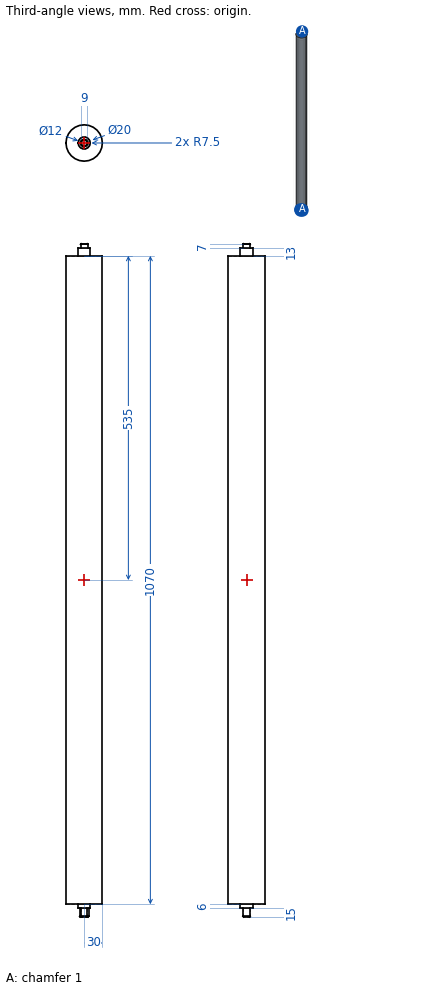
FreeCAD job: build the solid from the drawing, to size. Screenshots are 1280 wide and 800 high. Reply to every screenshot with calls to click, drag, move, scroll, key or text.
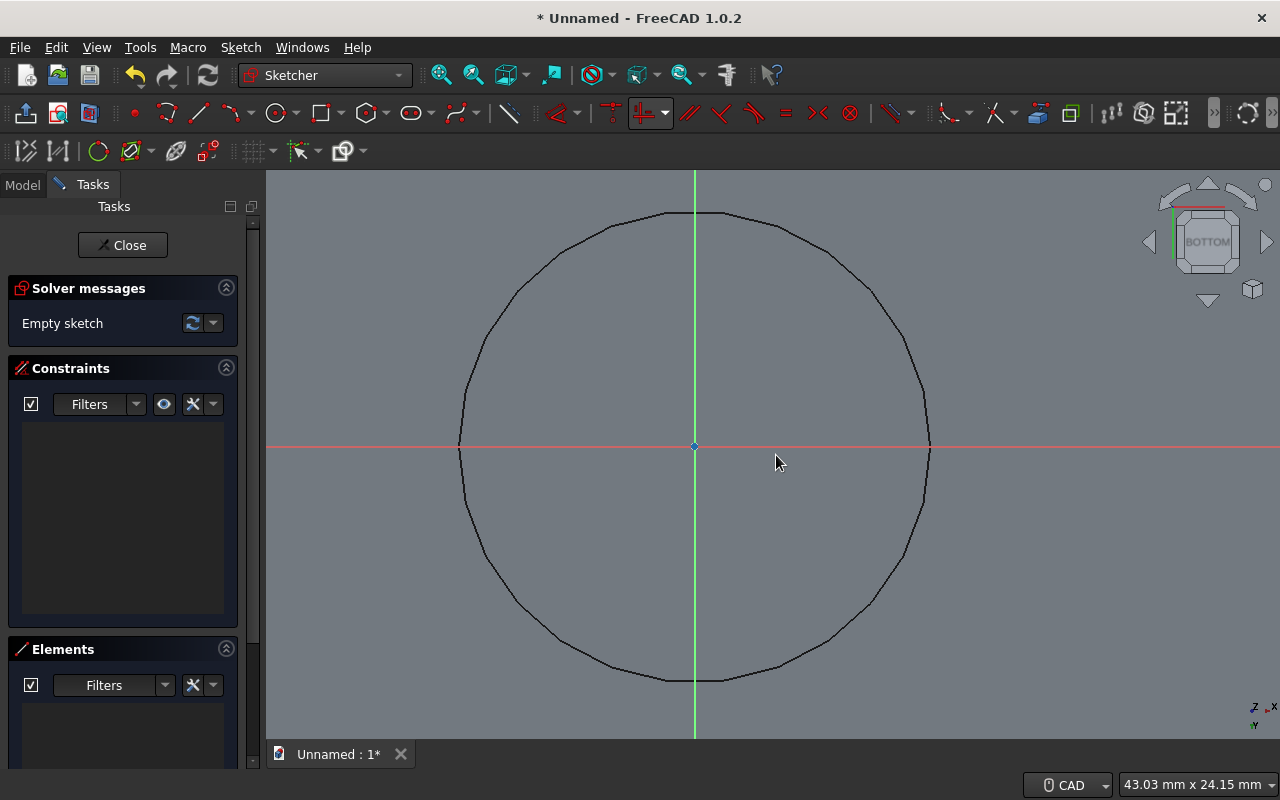
key(g)
key(l)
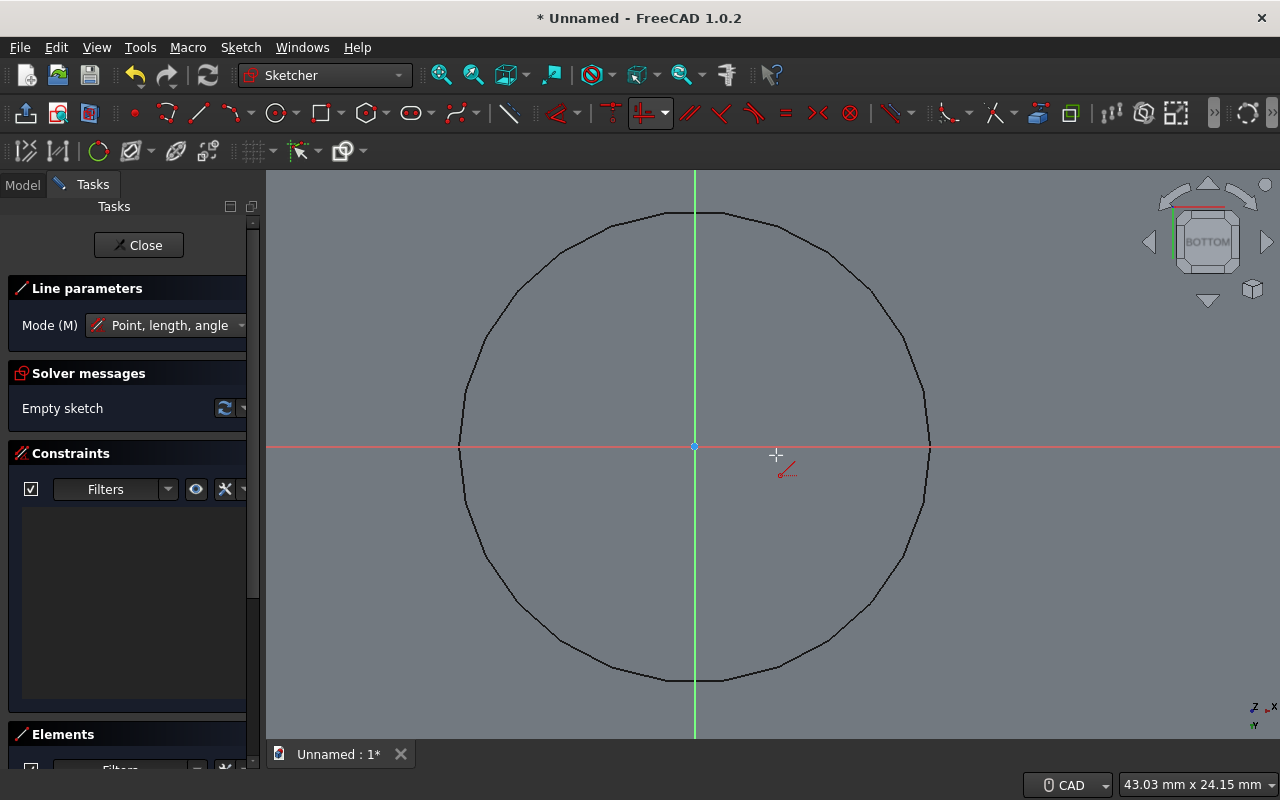
click(589, 588)
click(801, 588)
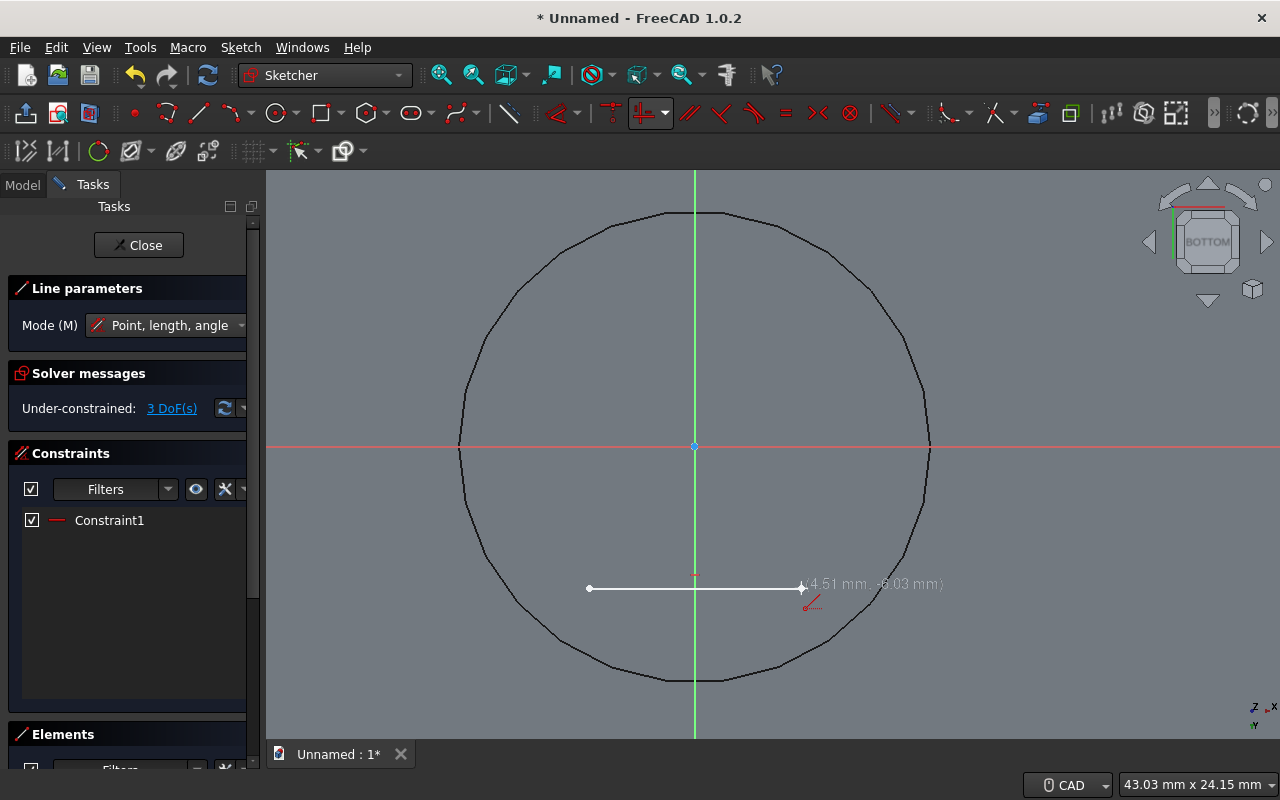
click(801, 306)
click(589, 306)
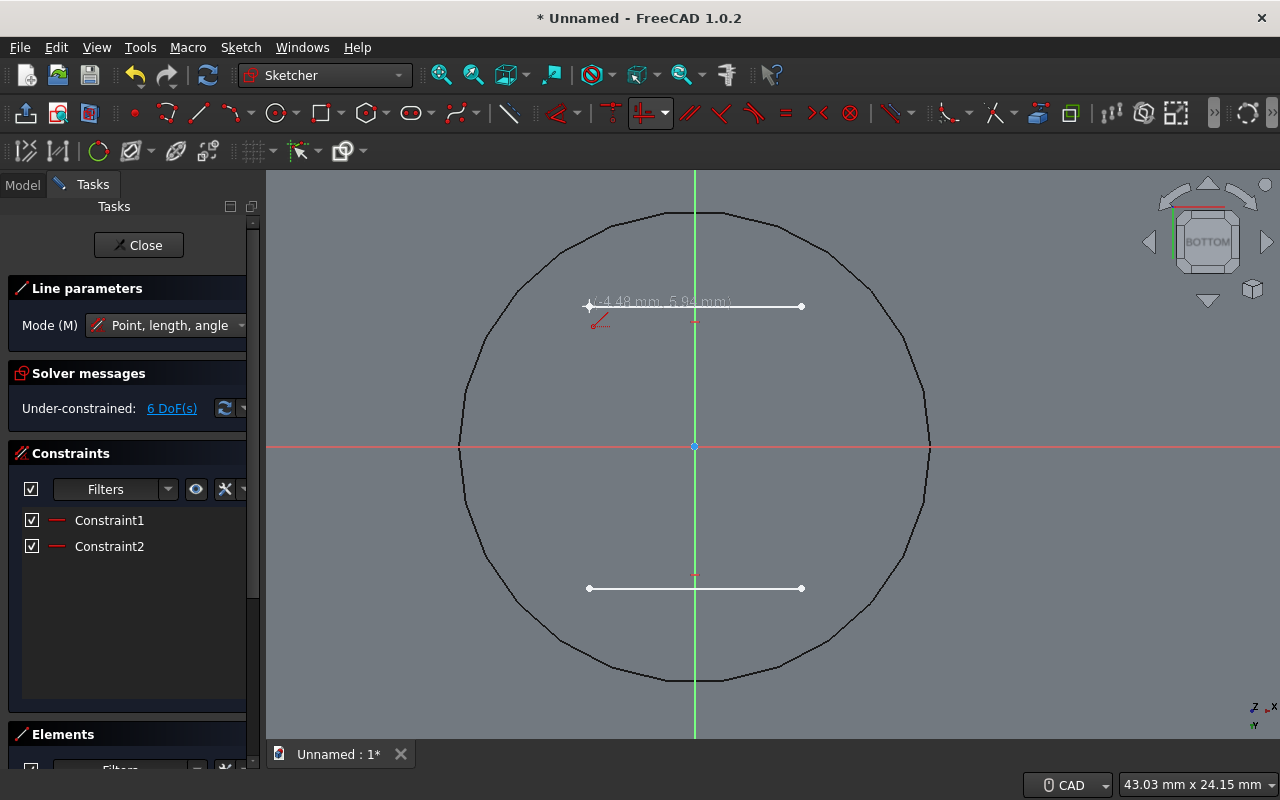
key(g)
key(3)
key(a)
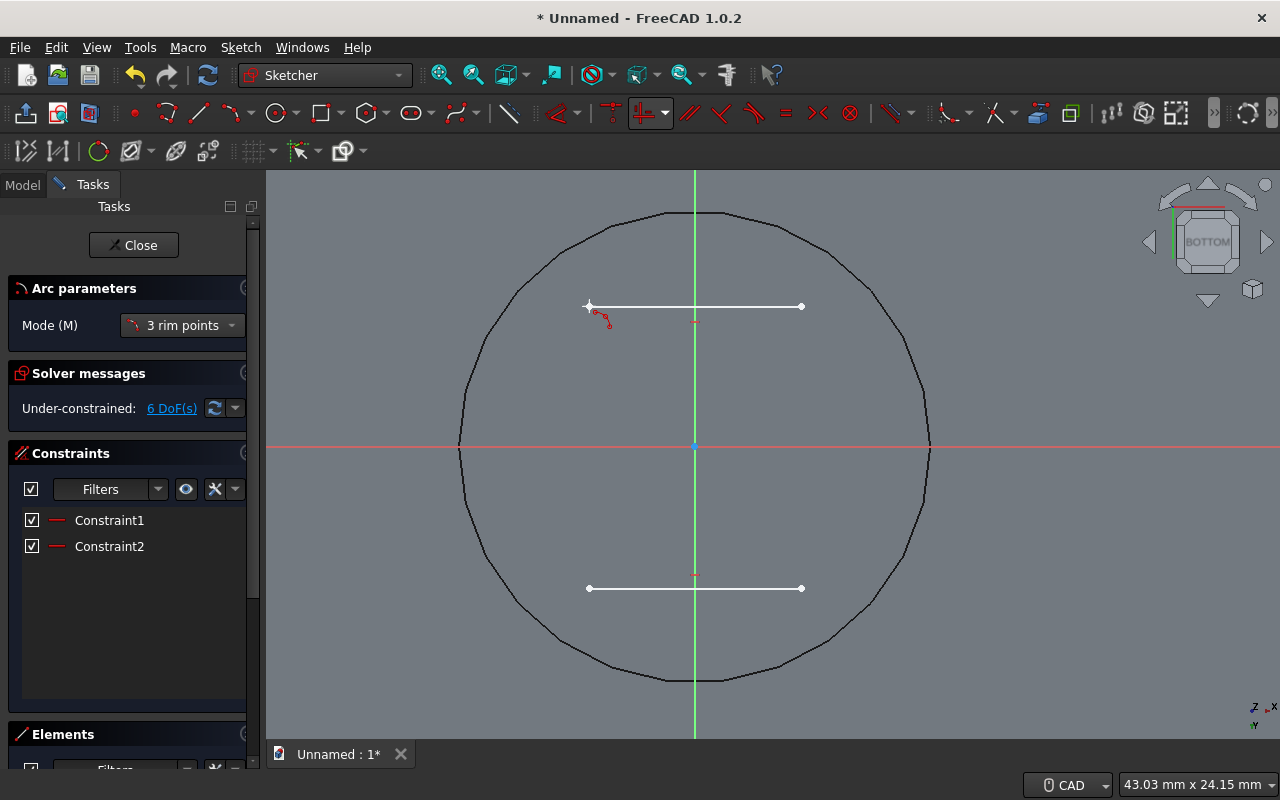
click(801, 589)
click(801, 307)
click(868, 480)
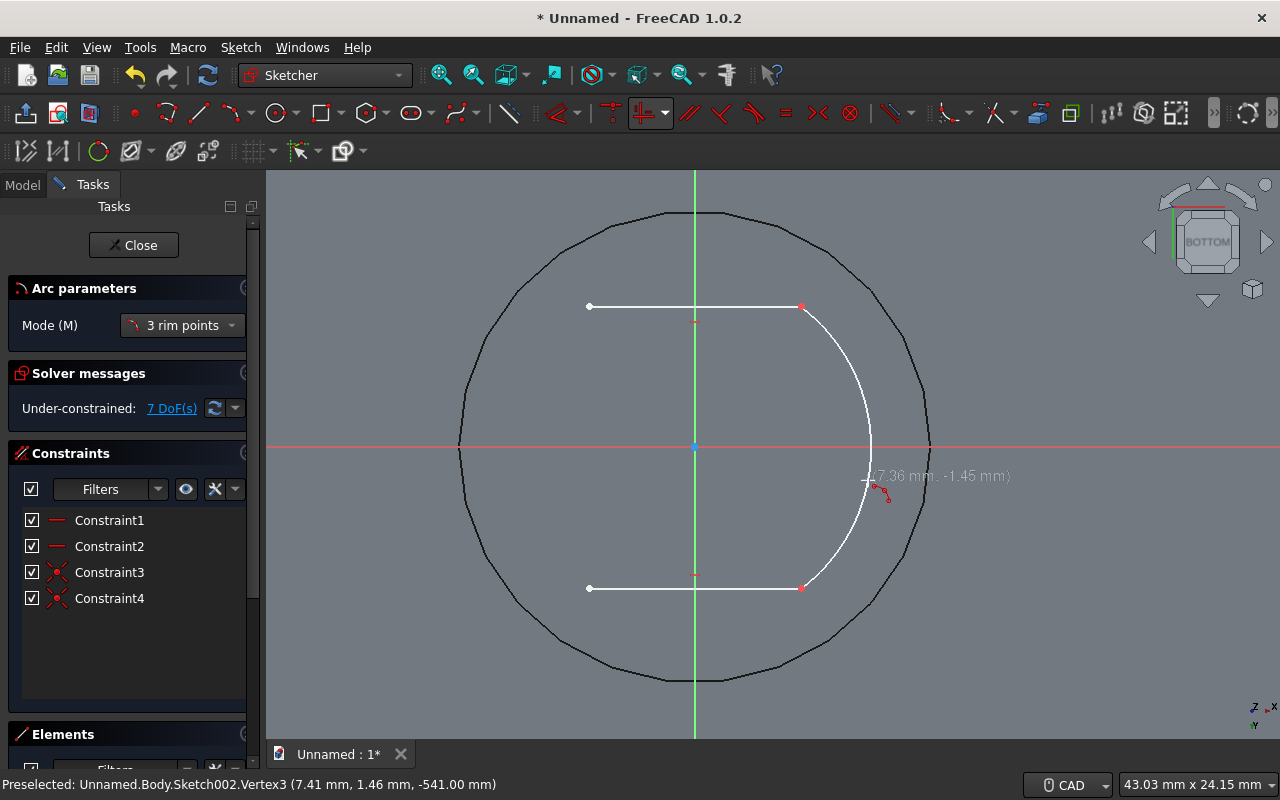
click(589, 307)
click(589, 589)
click(521, 414)
key(Escape)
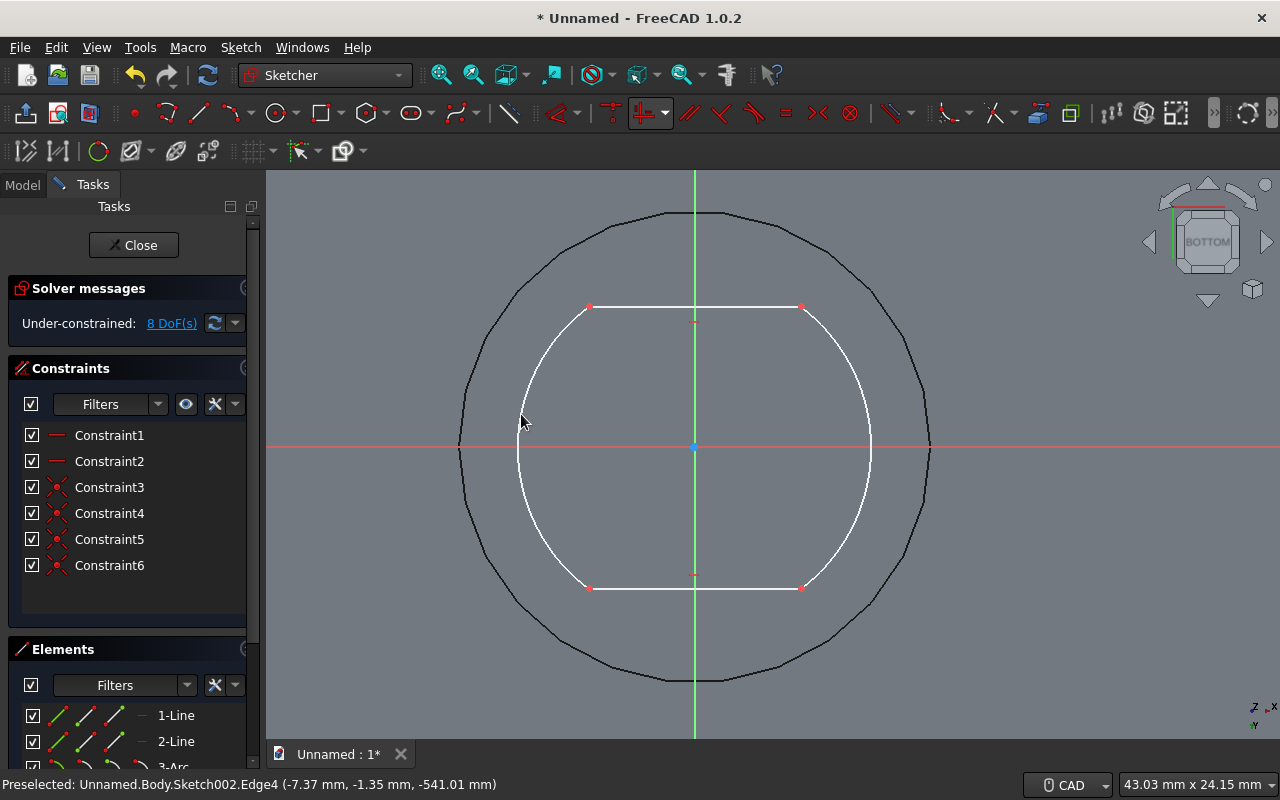
click(859, 512)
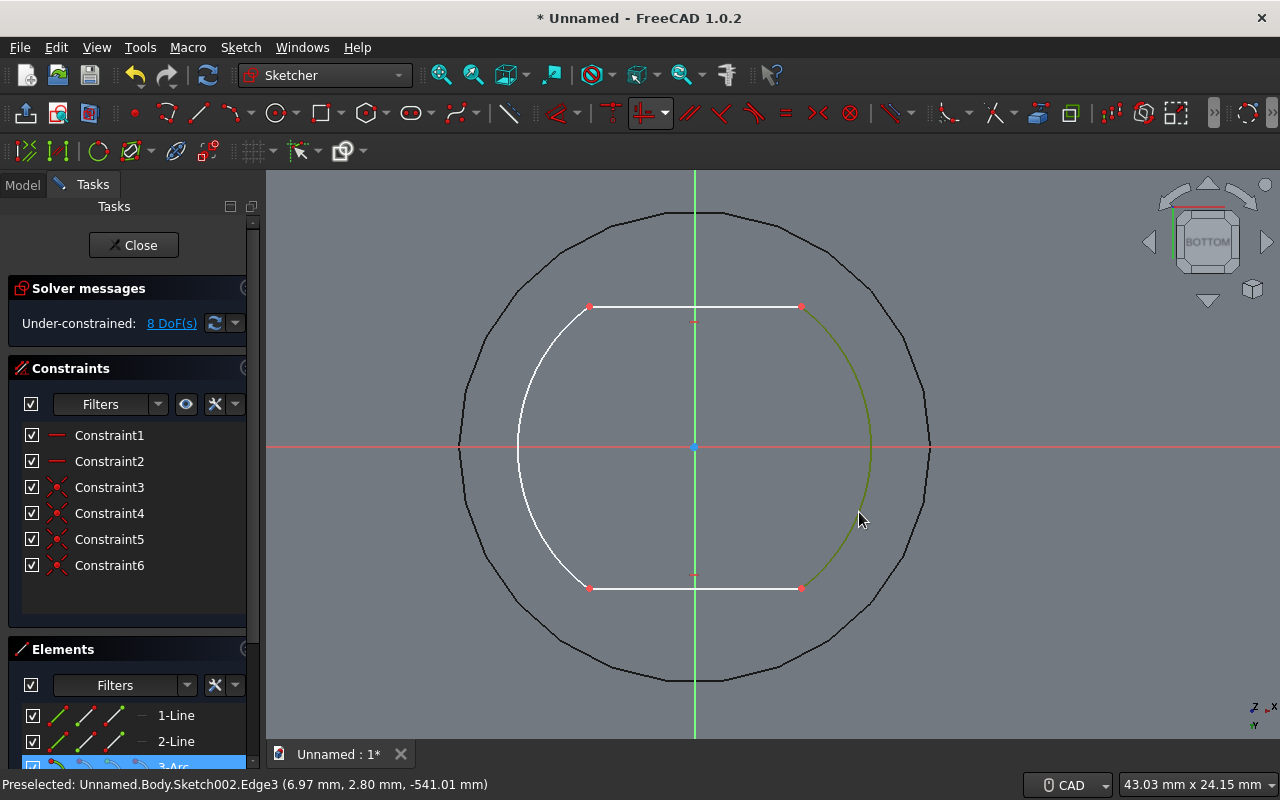
click(530, 384)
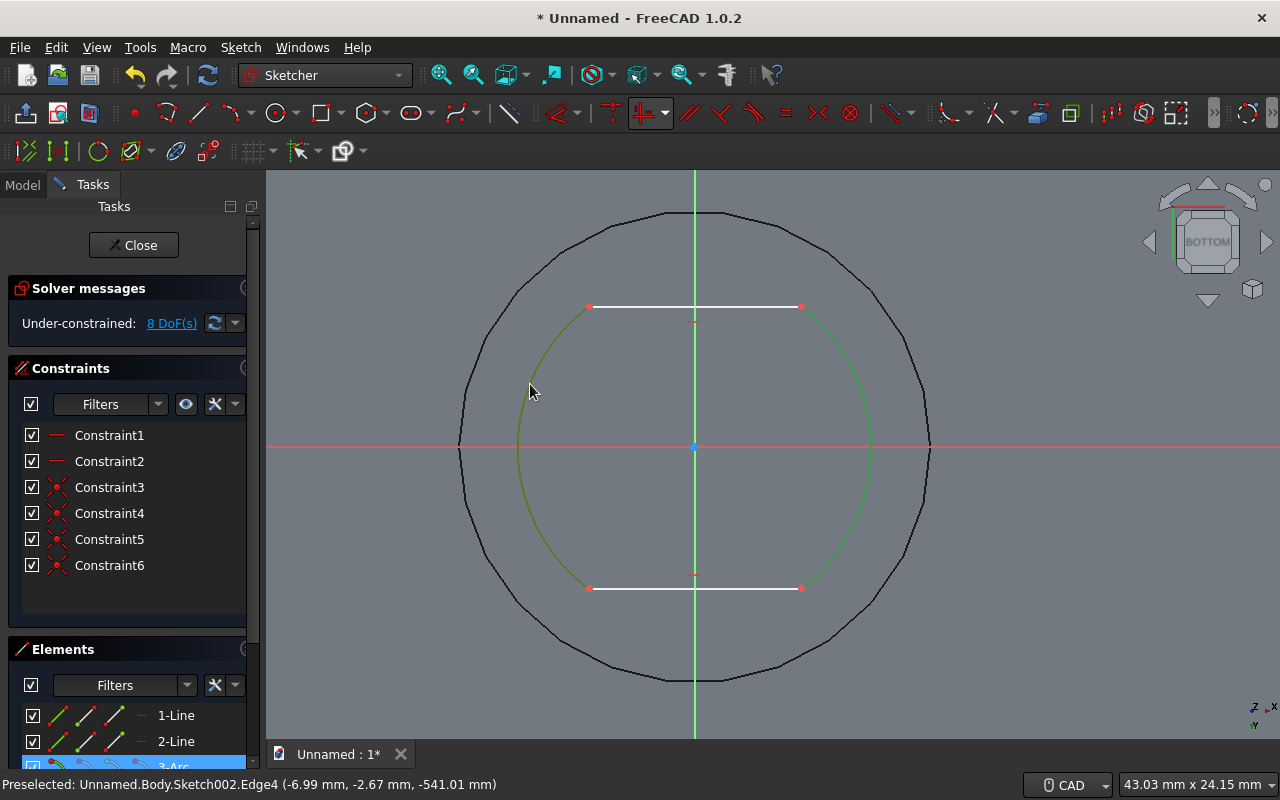
click(612, 114)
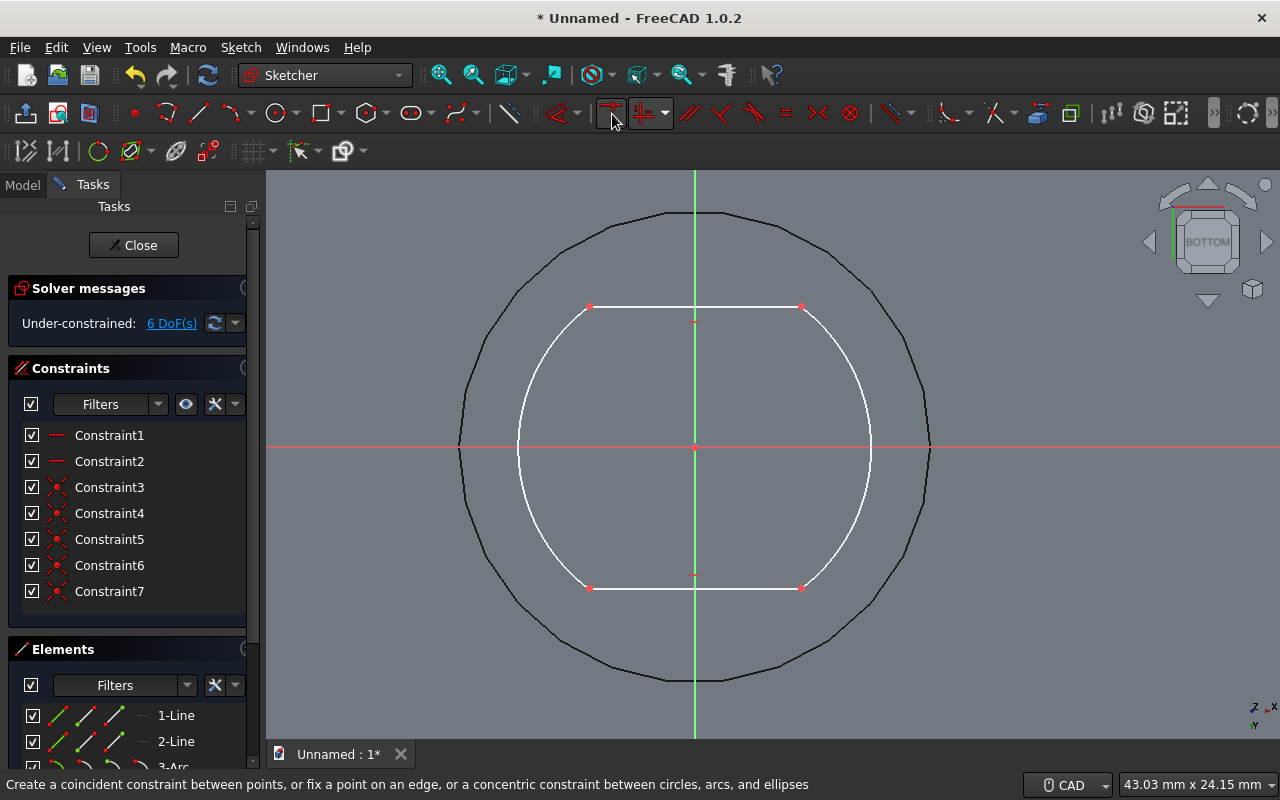
drag(684, 437, 705, 458)